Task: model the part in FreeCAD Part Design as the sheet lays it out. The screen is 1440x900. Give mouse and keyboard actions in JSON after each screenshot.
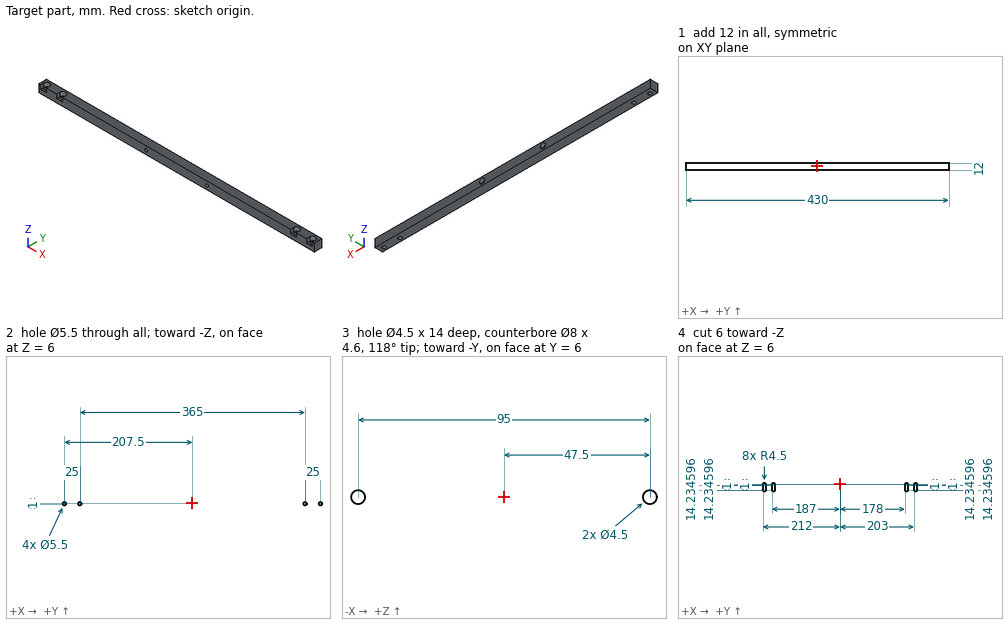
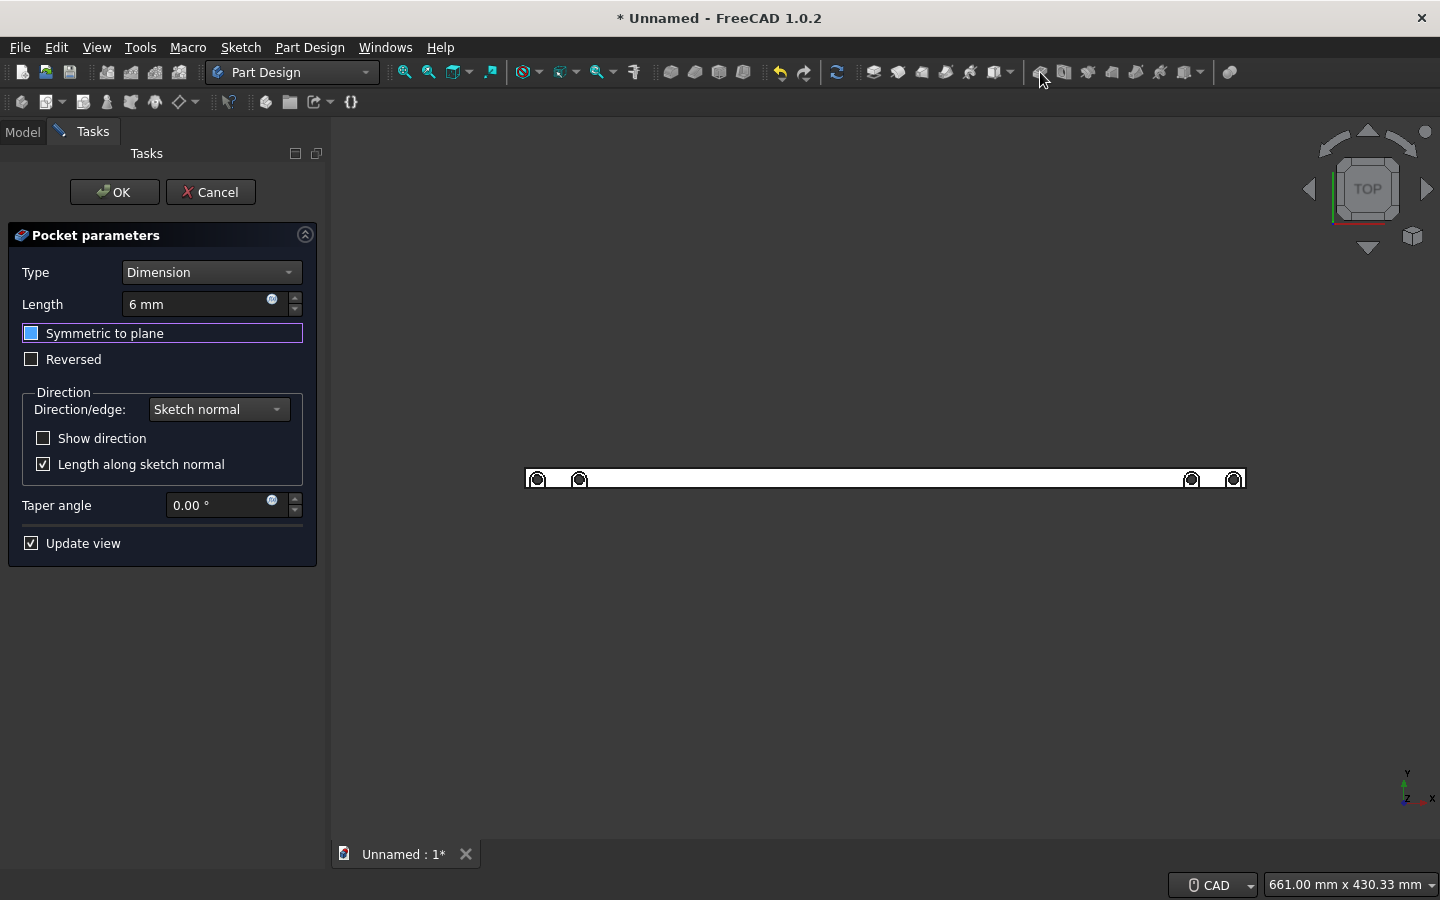
{"action": "left_click", "coordinate": [115, 192]}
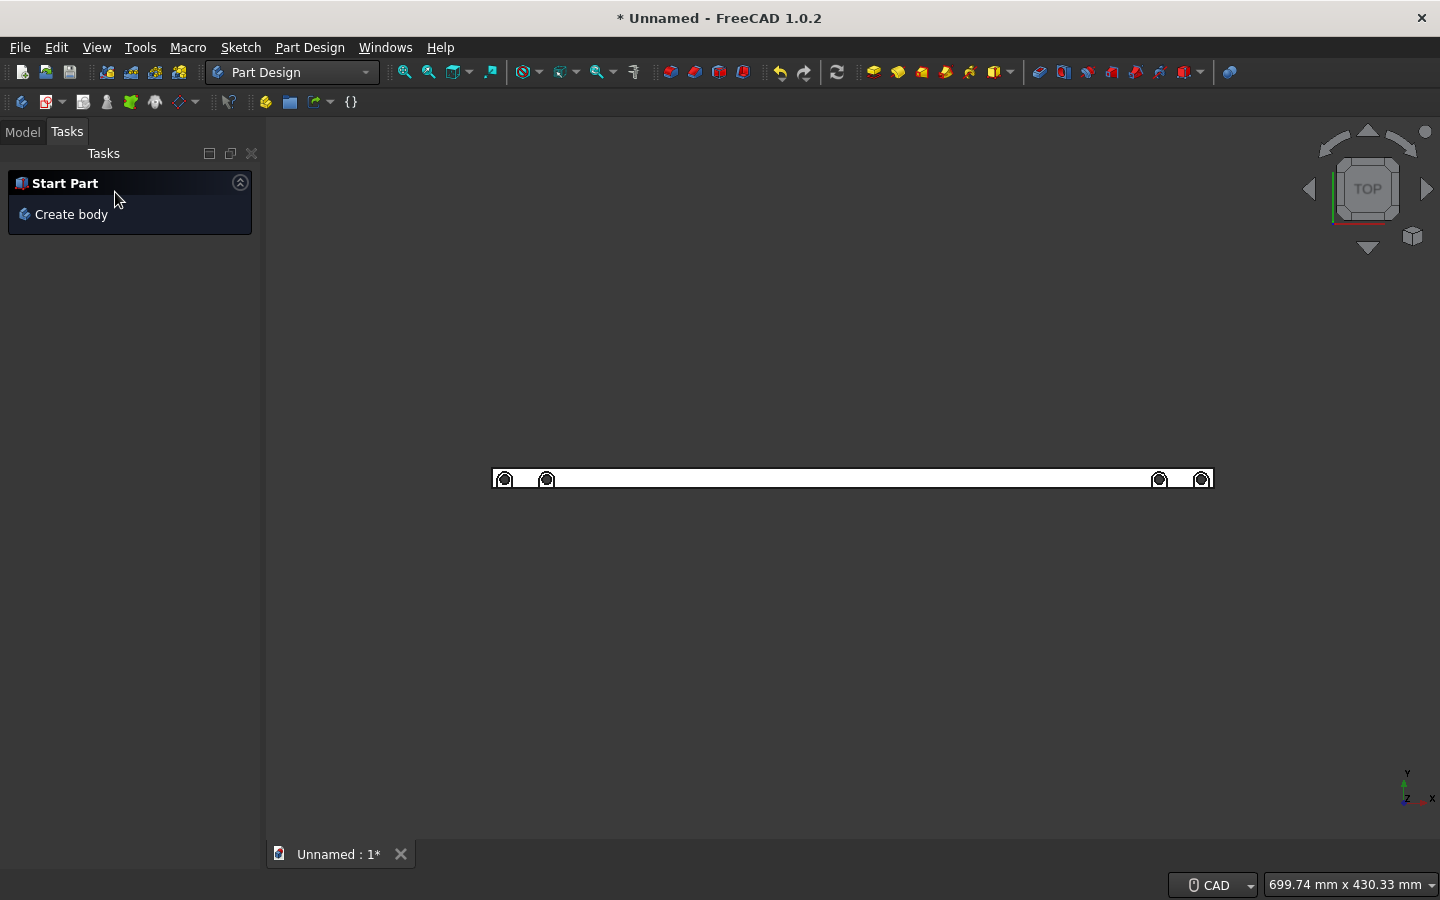
{"action": "key", "text": "0"}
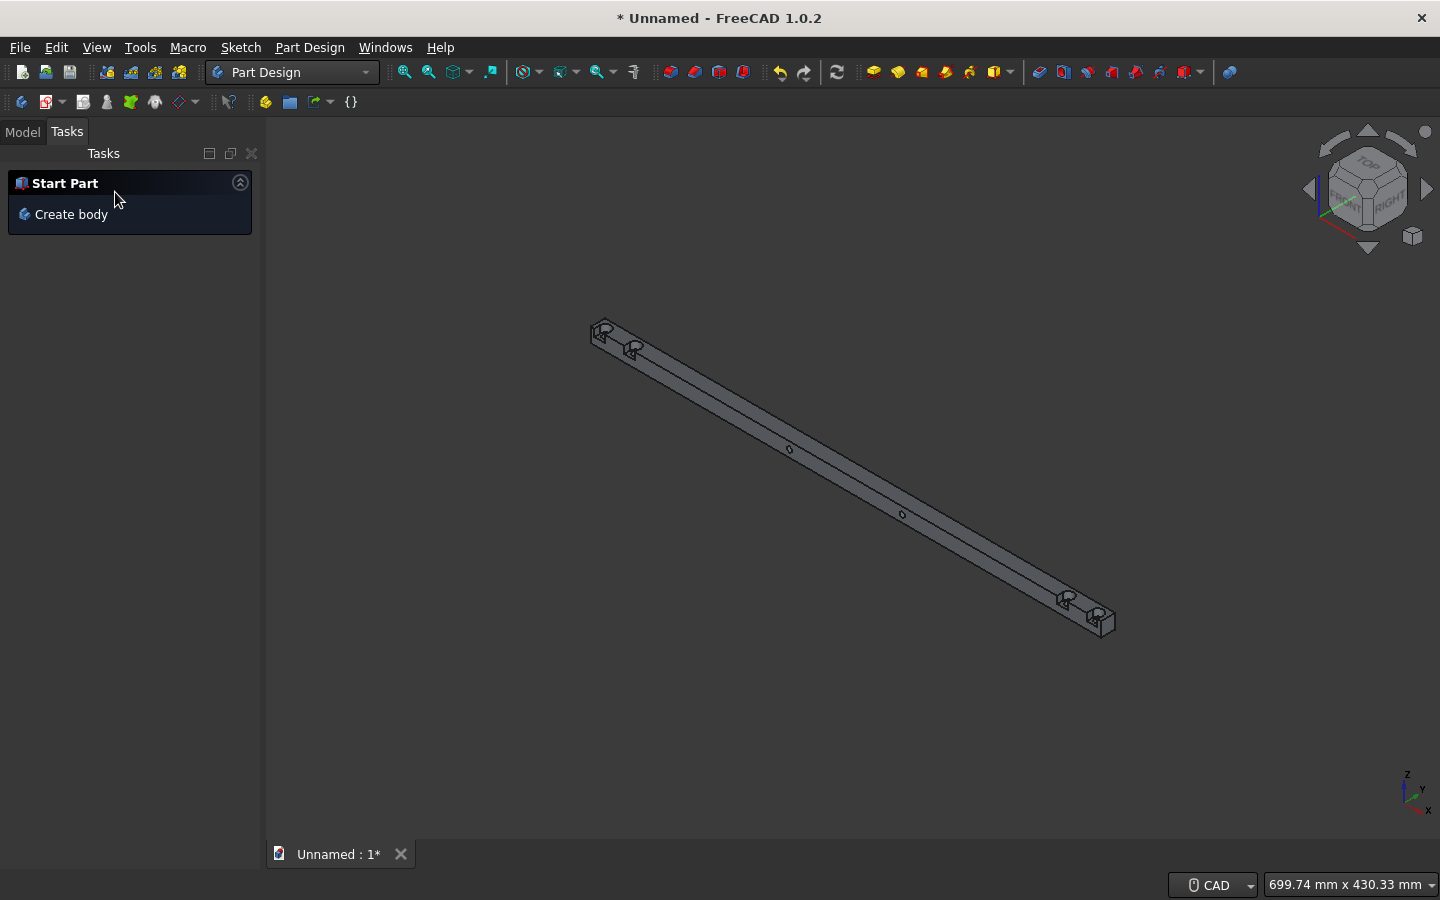
{"action": "left_click", "coordinate": [406, 72]}